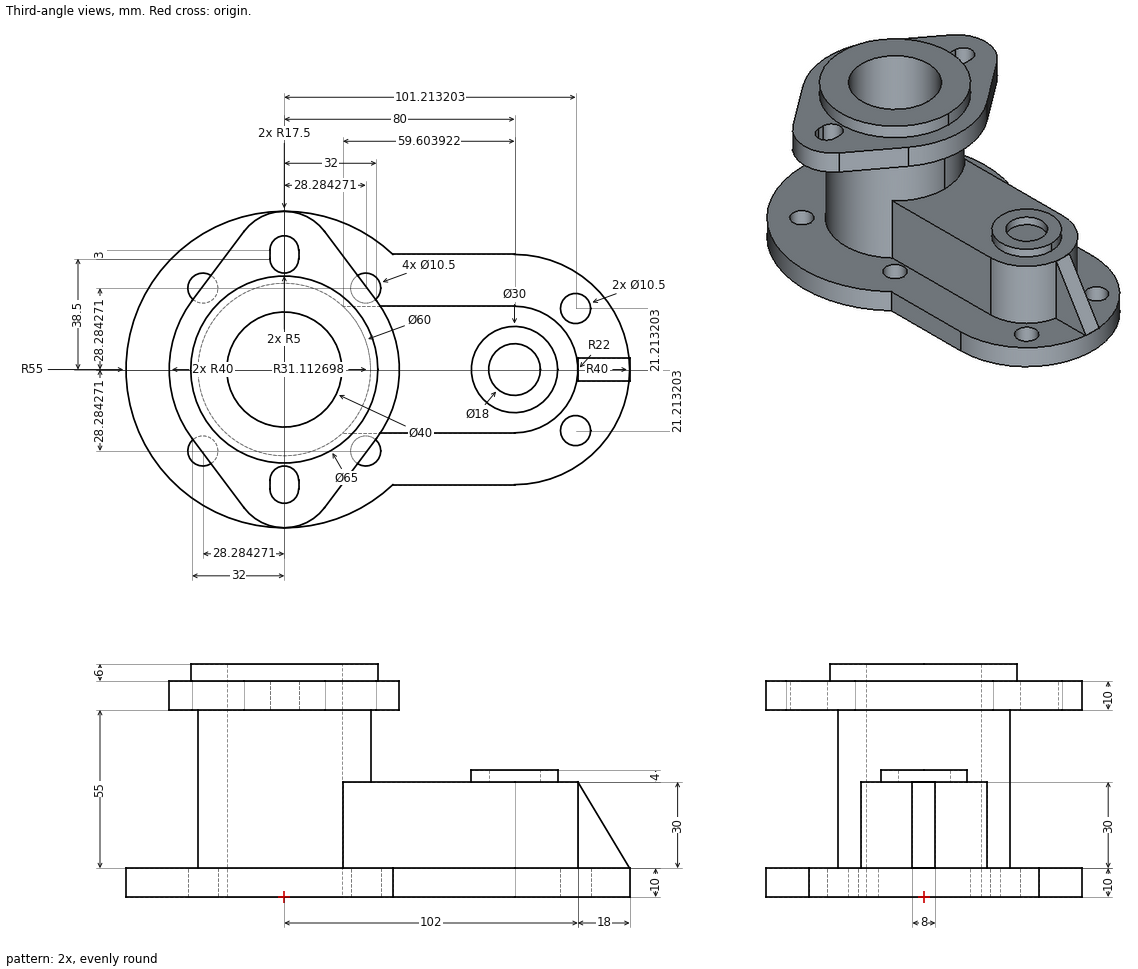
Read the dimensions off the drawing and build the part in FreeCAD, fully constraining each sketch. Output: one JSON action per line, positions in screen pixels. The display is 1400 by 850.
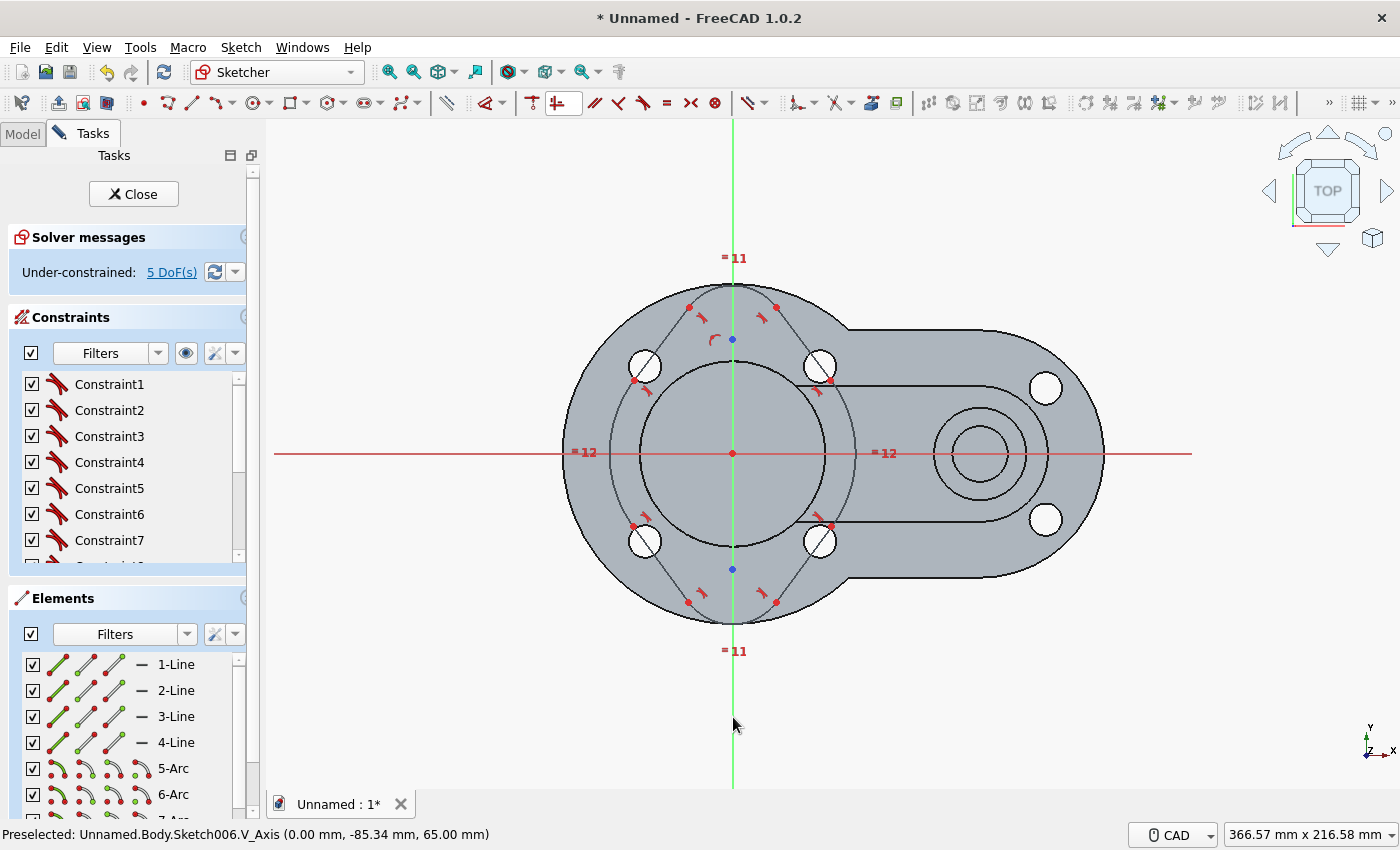
{"action": "left_click", "coordinate": [733, 570]}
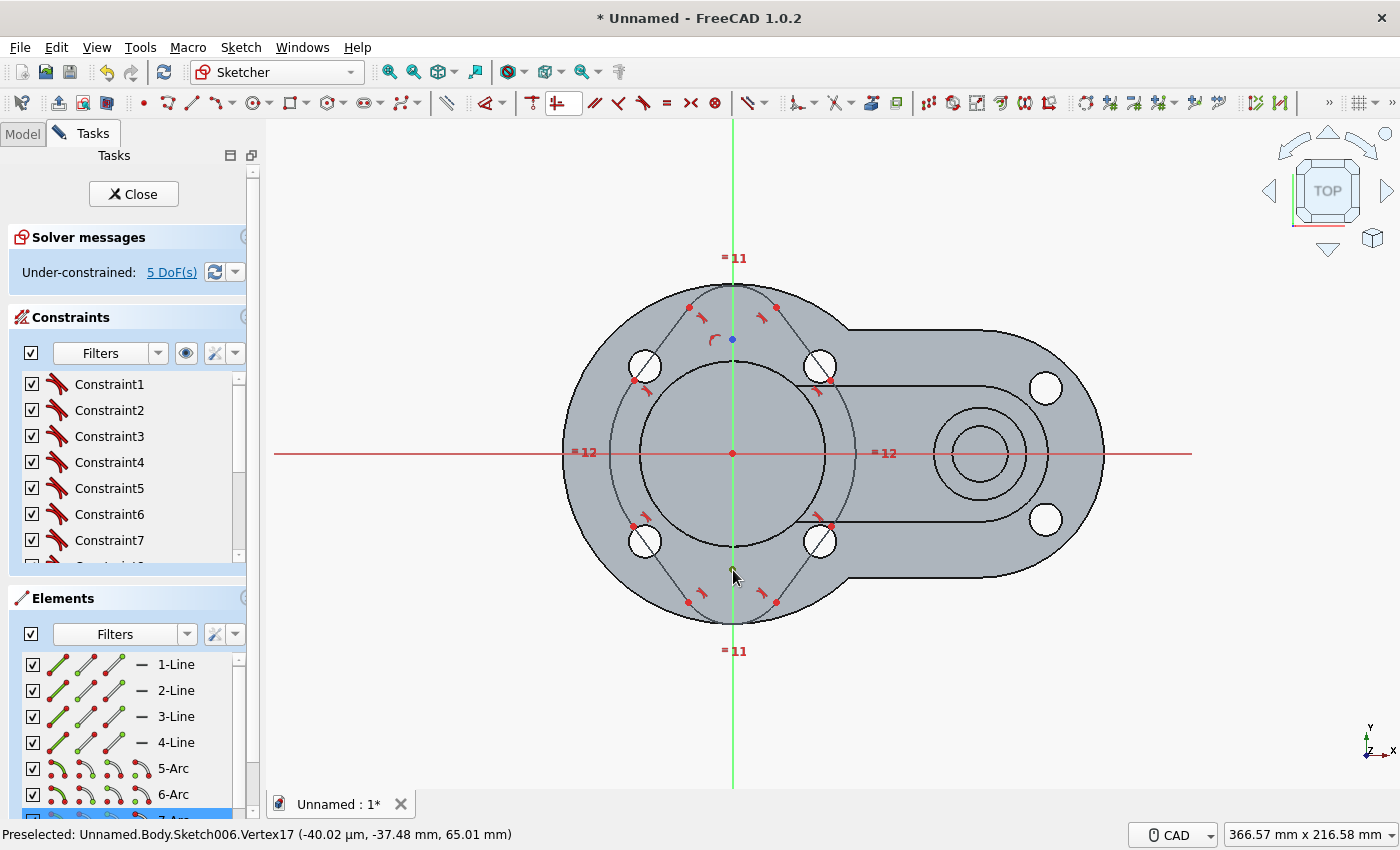
{"action": "left_click", "coordinate": [733, 717]}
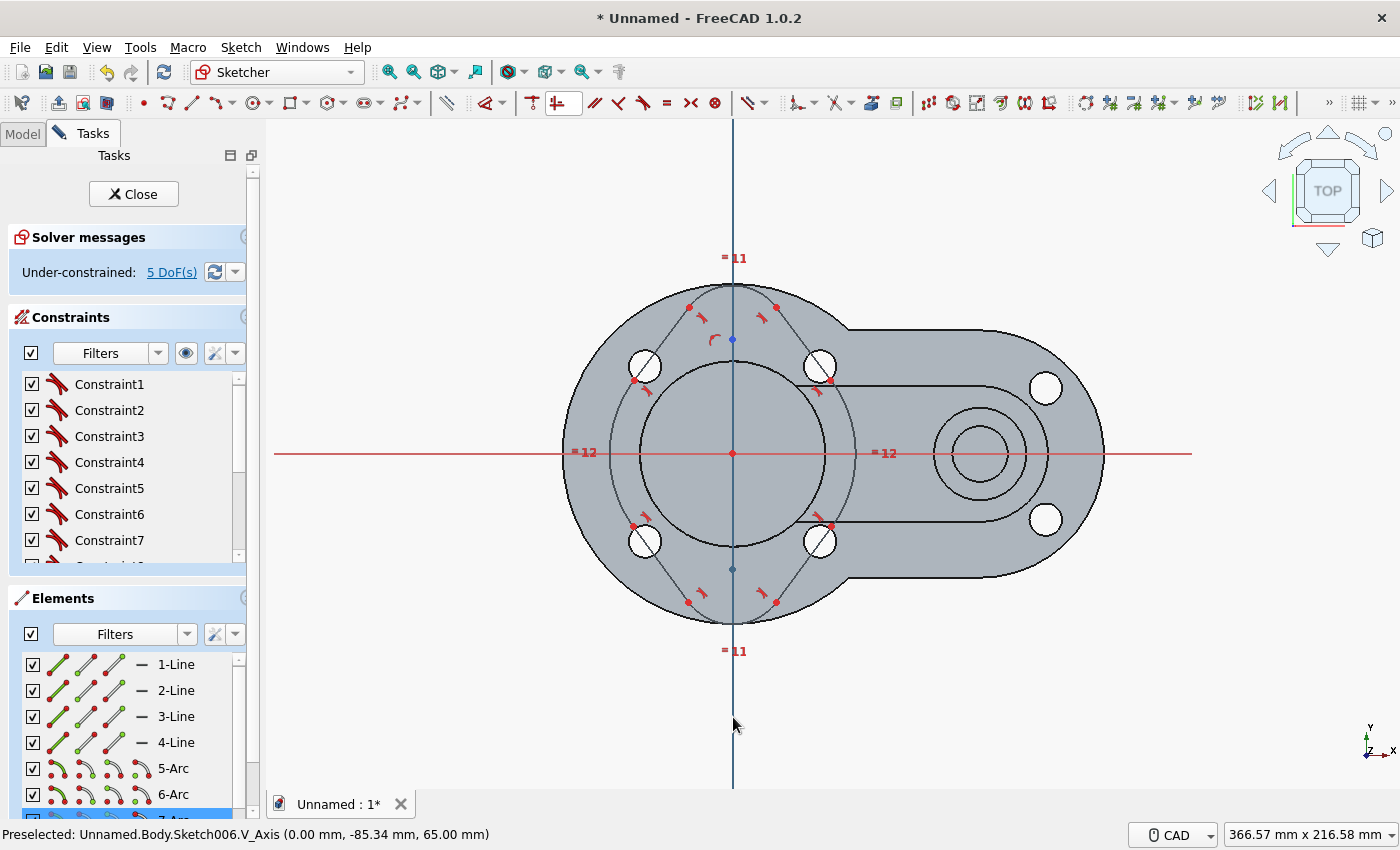
{"action": "key", "text": "c"}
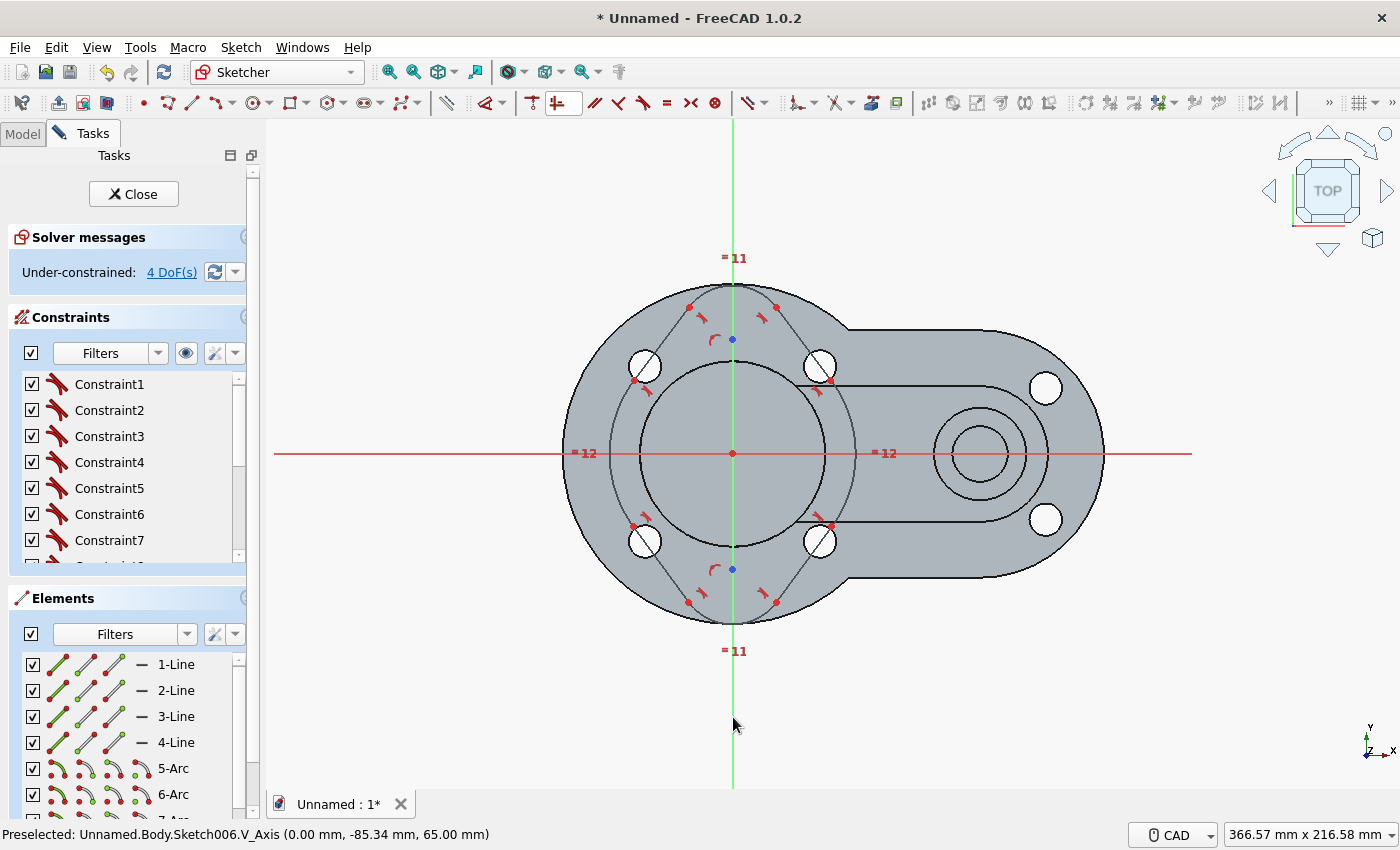
{"action": "left_click", "coordinate": [486, 104]}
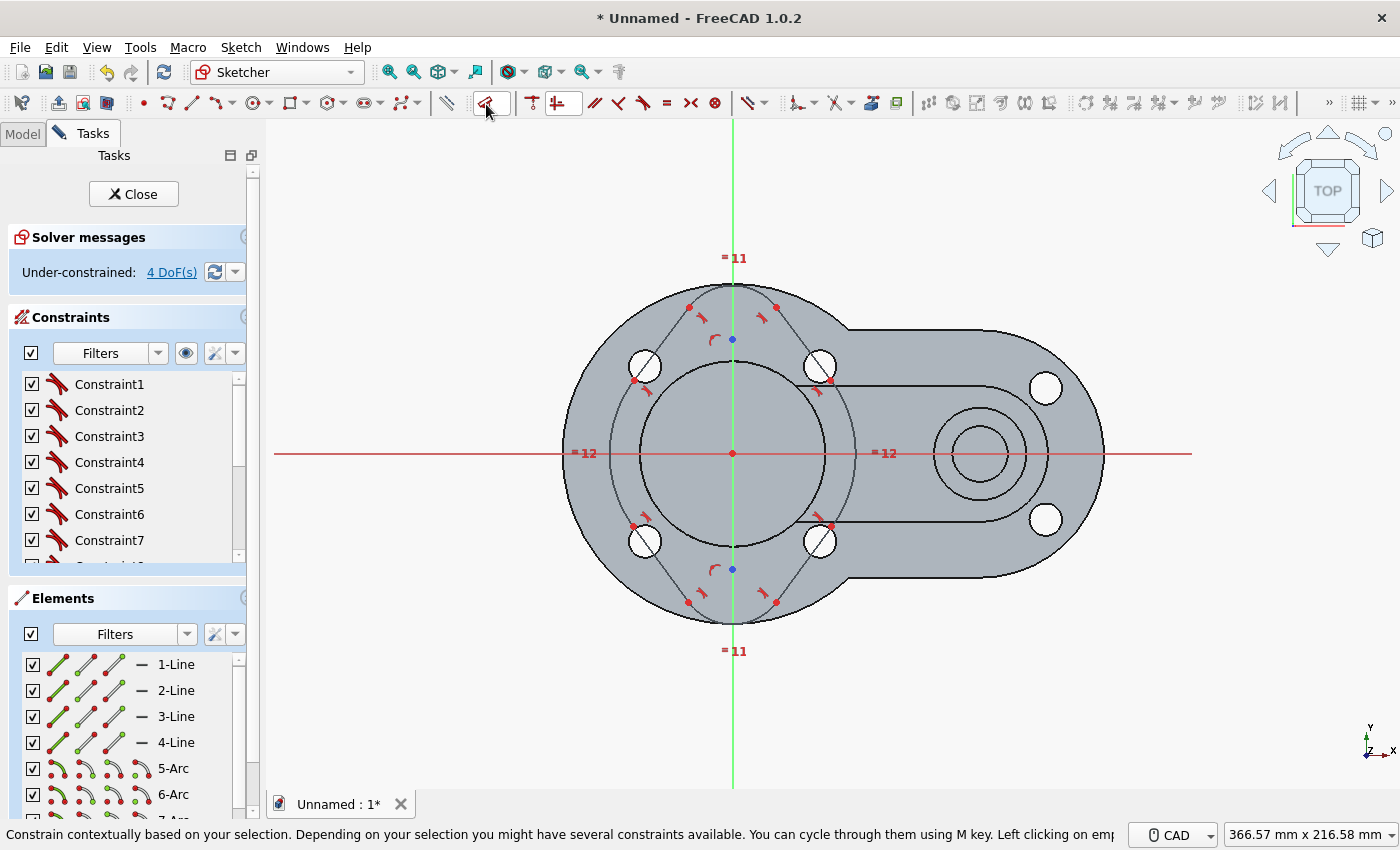
{"action": "left_click", "coordinate": [752, 289]}
{"action": "left_click", "coordinate": [763, 259]}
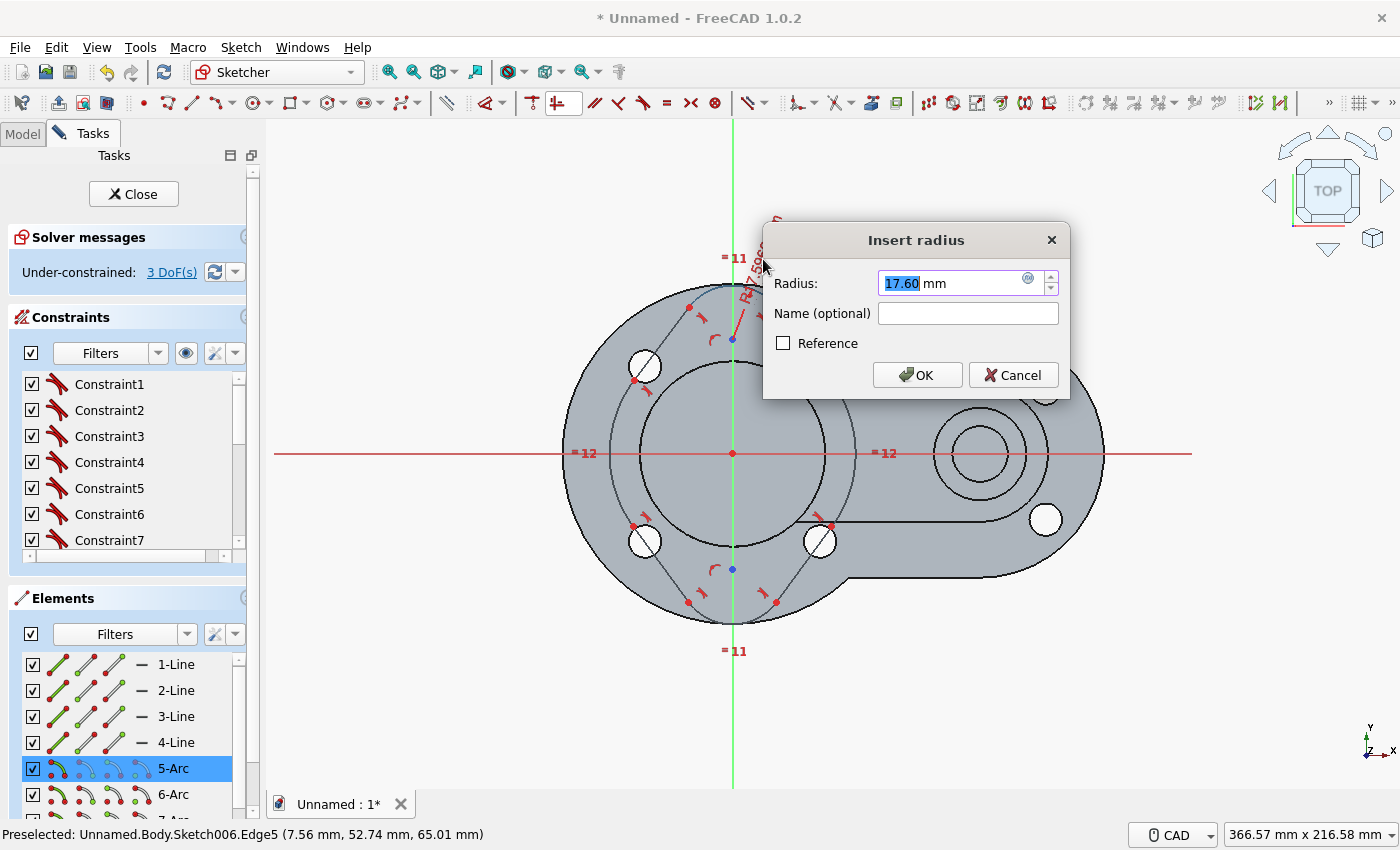
{"action": "type", "text": "17.5"}
{"action": "key", "text": "Return"}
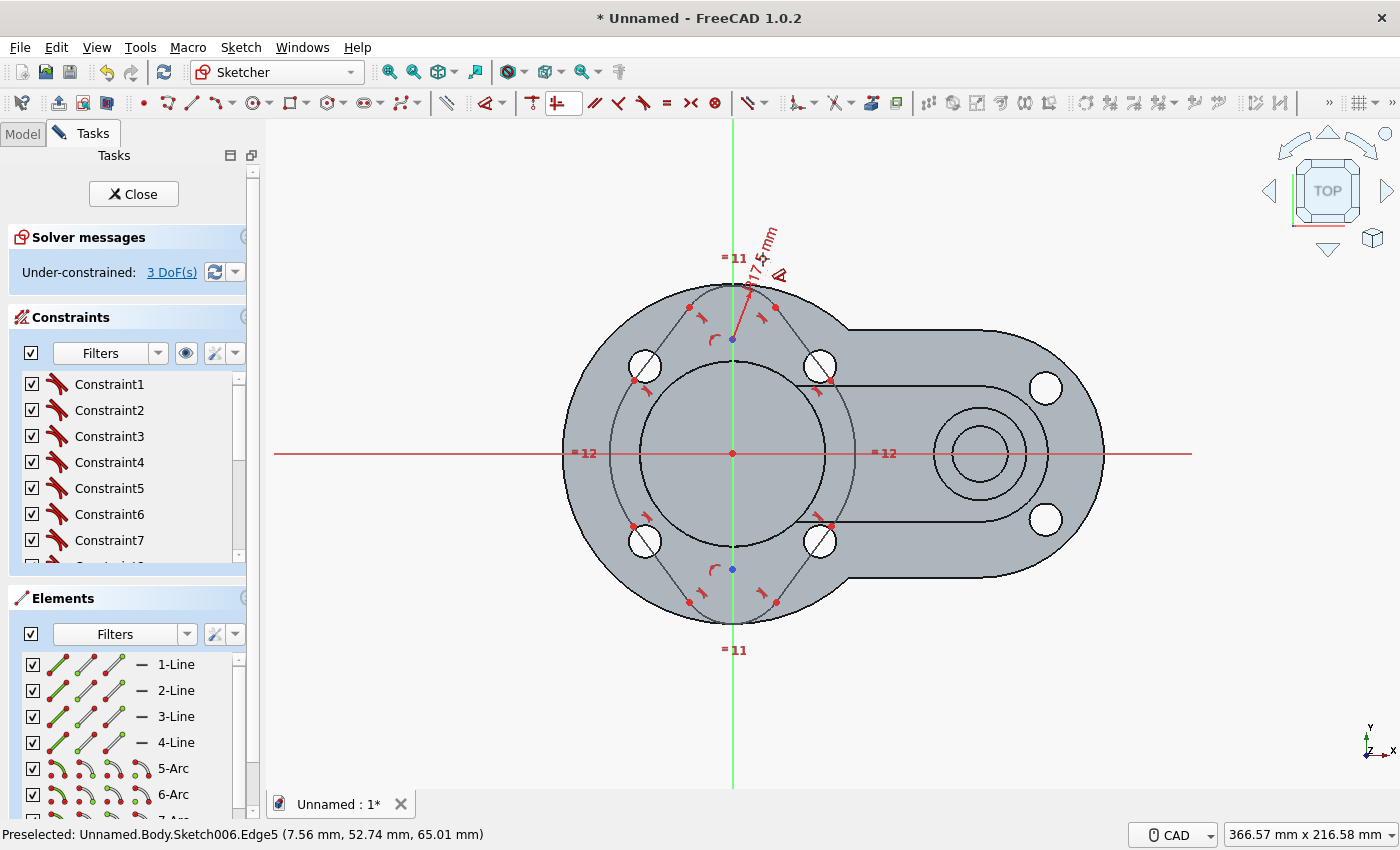
{"action": "left_click", "coordinate": [614, 422]}
{"action": "left_click", "coordinate": [583, 414]}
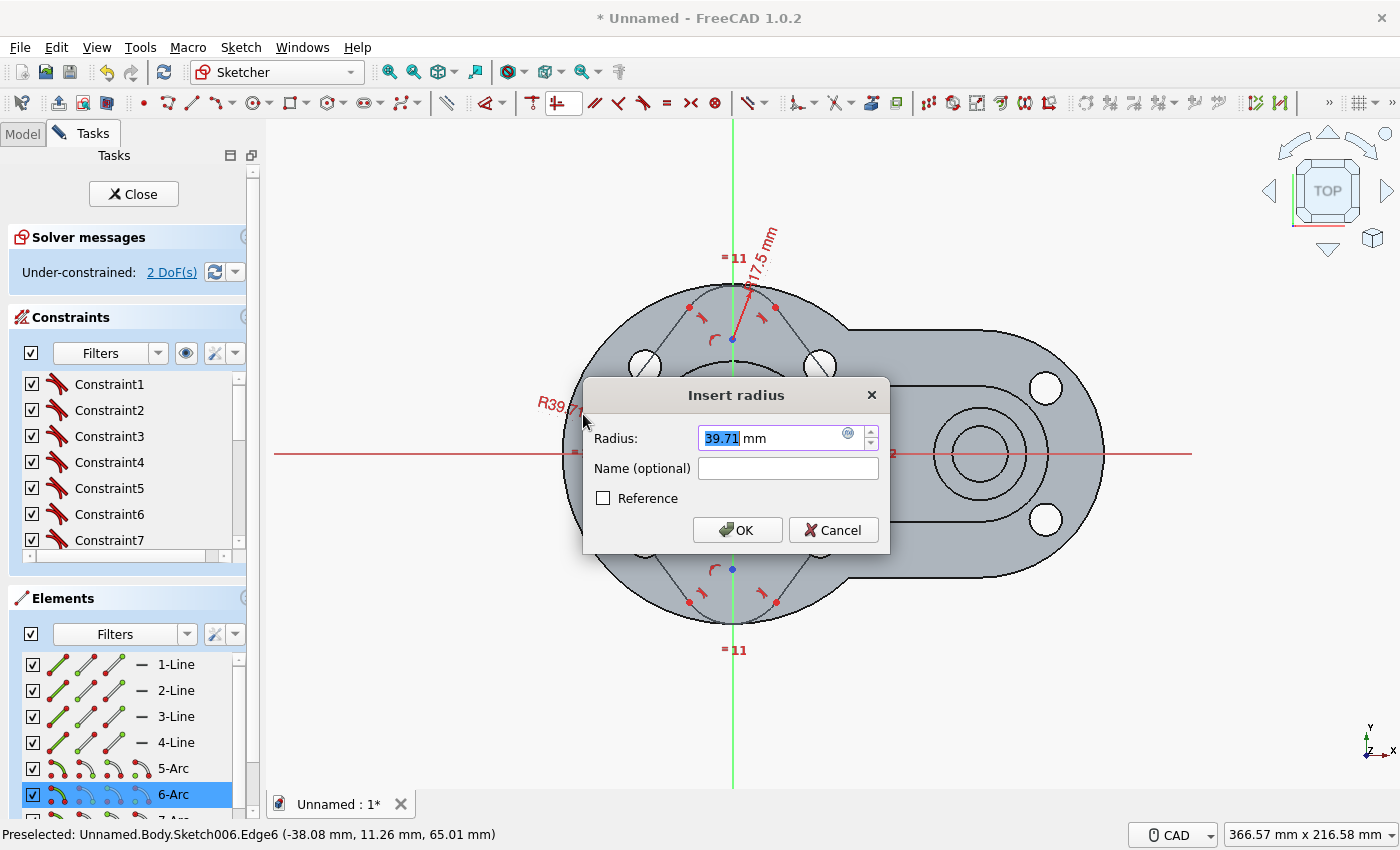
{"action": "type", "text": "40"}
{"action": "key", "text": "Return"}